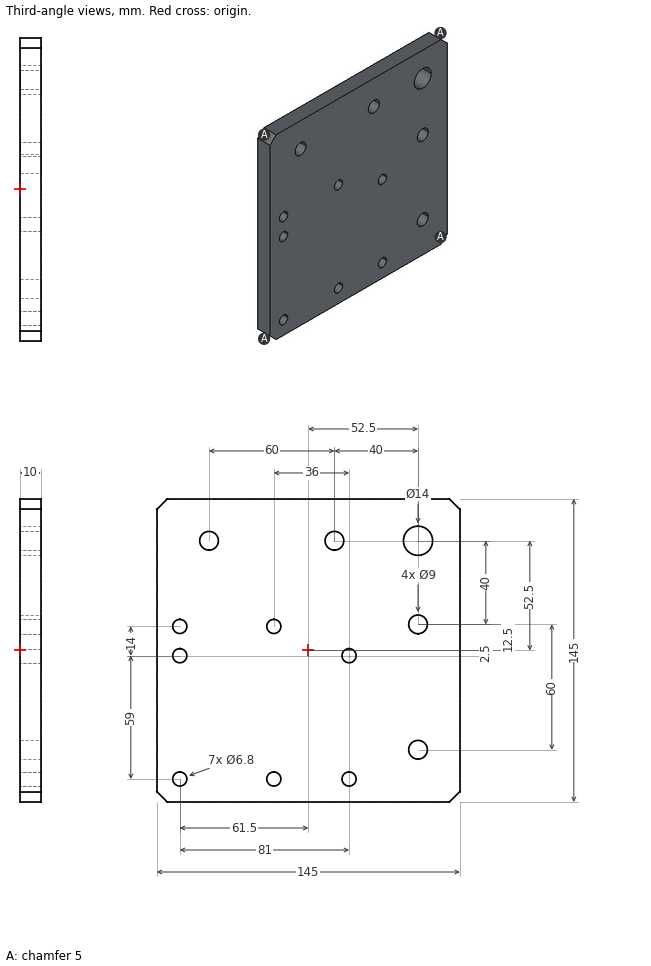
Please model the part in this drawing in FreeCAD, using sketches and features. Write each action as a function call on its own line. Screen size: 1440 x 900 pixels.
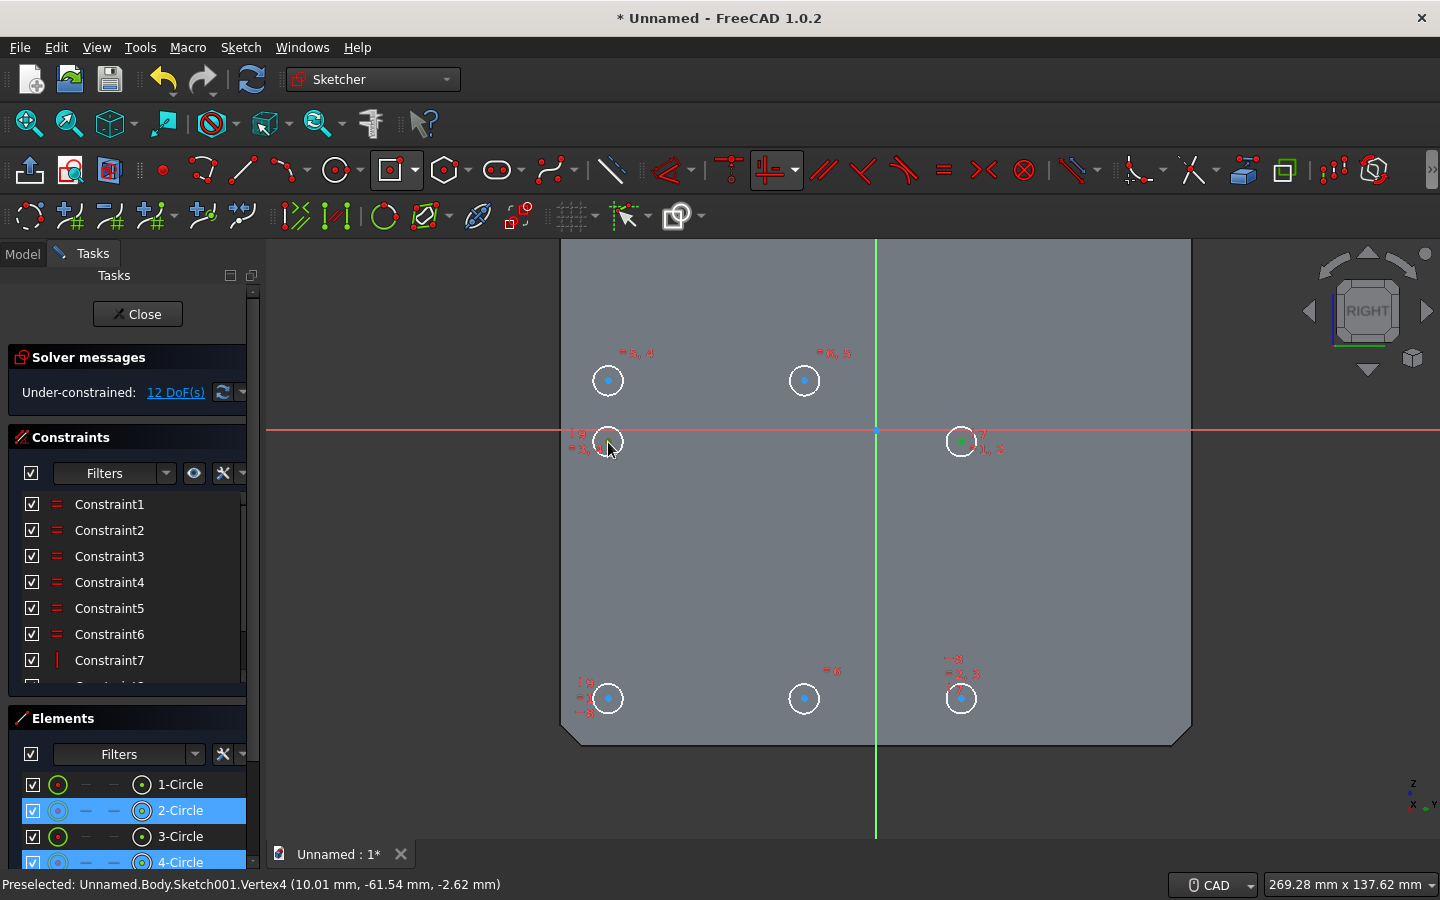
click(798, 170)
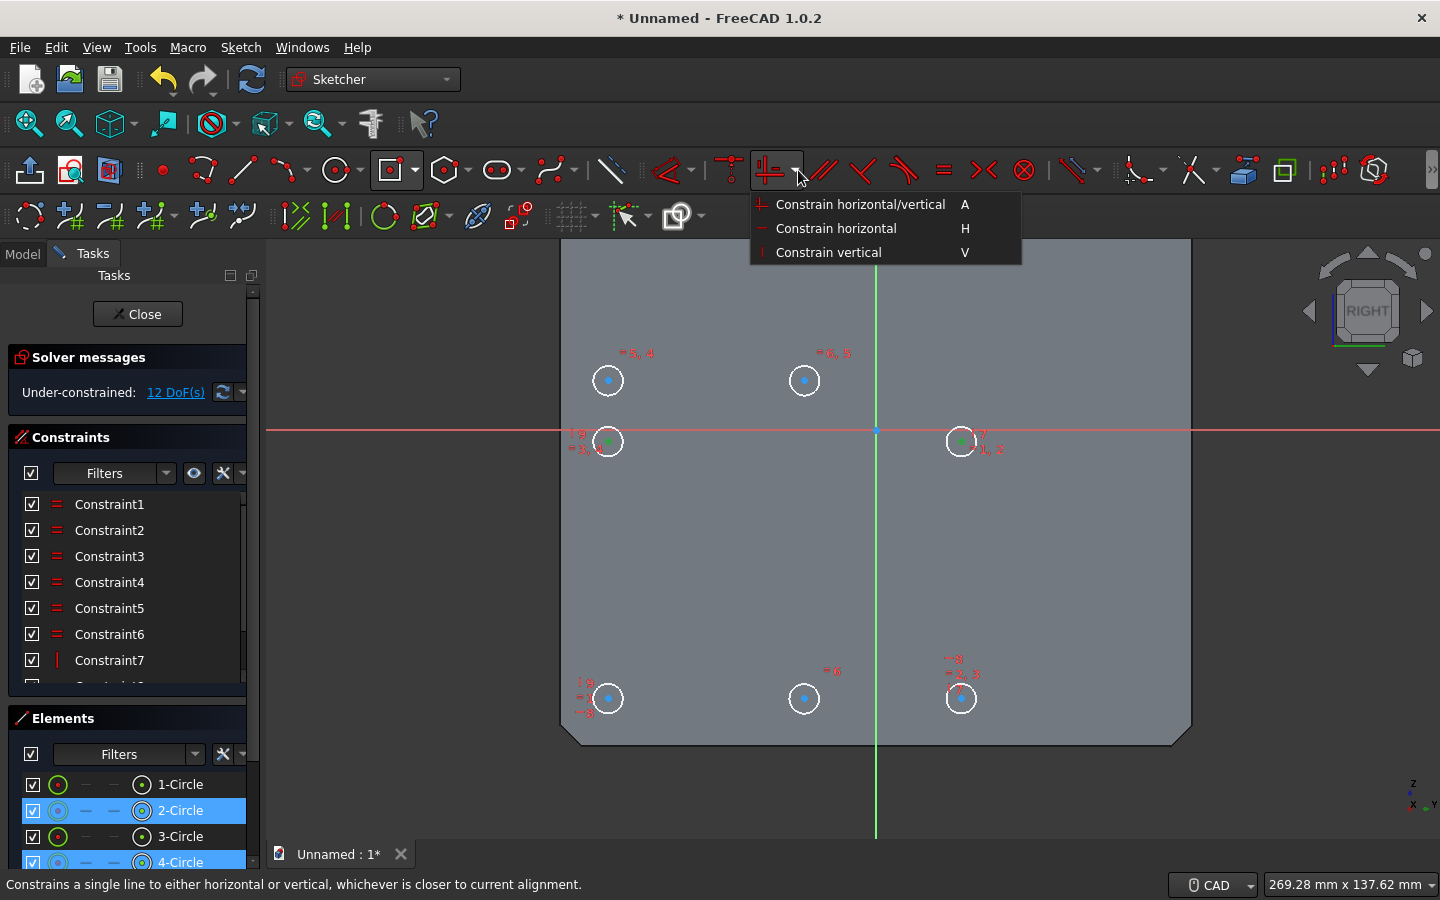
click(886, 228)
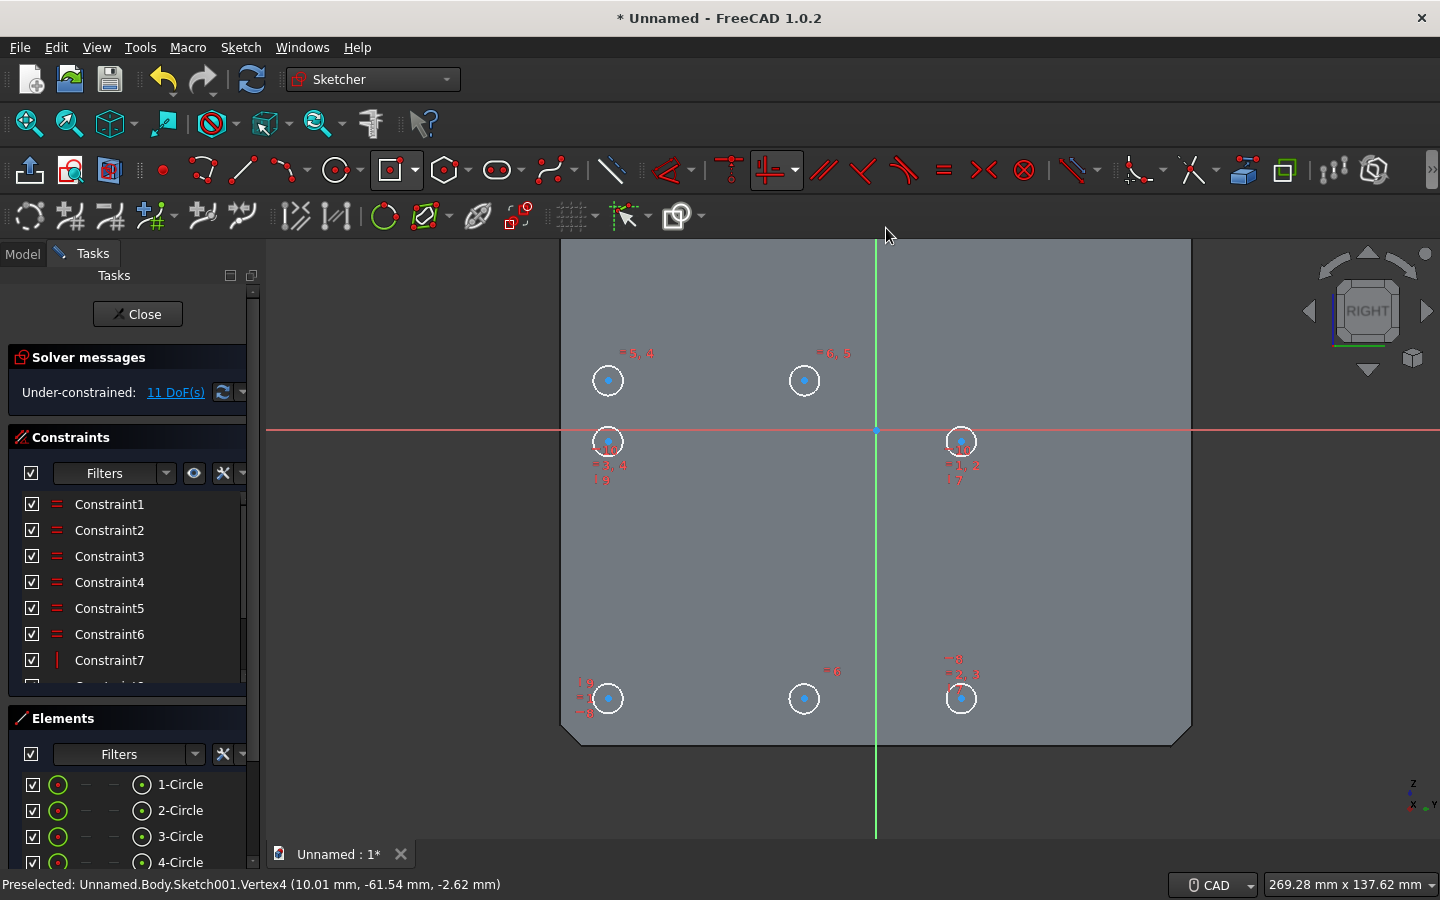
click(608, 442)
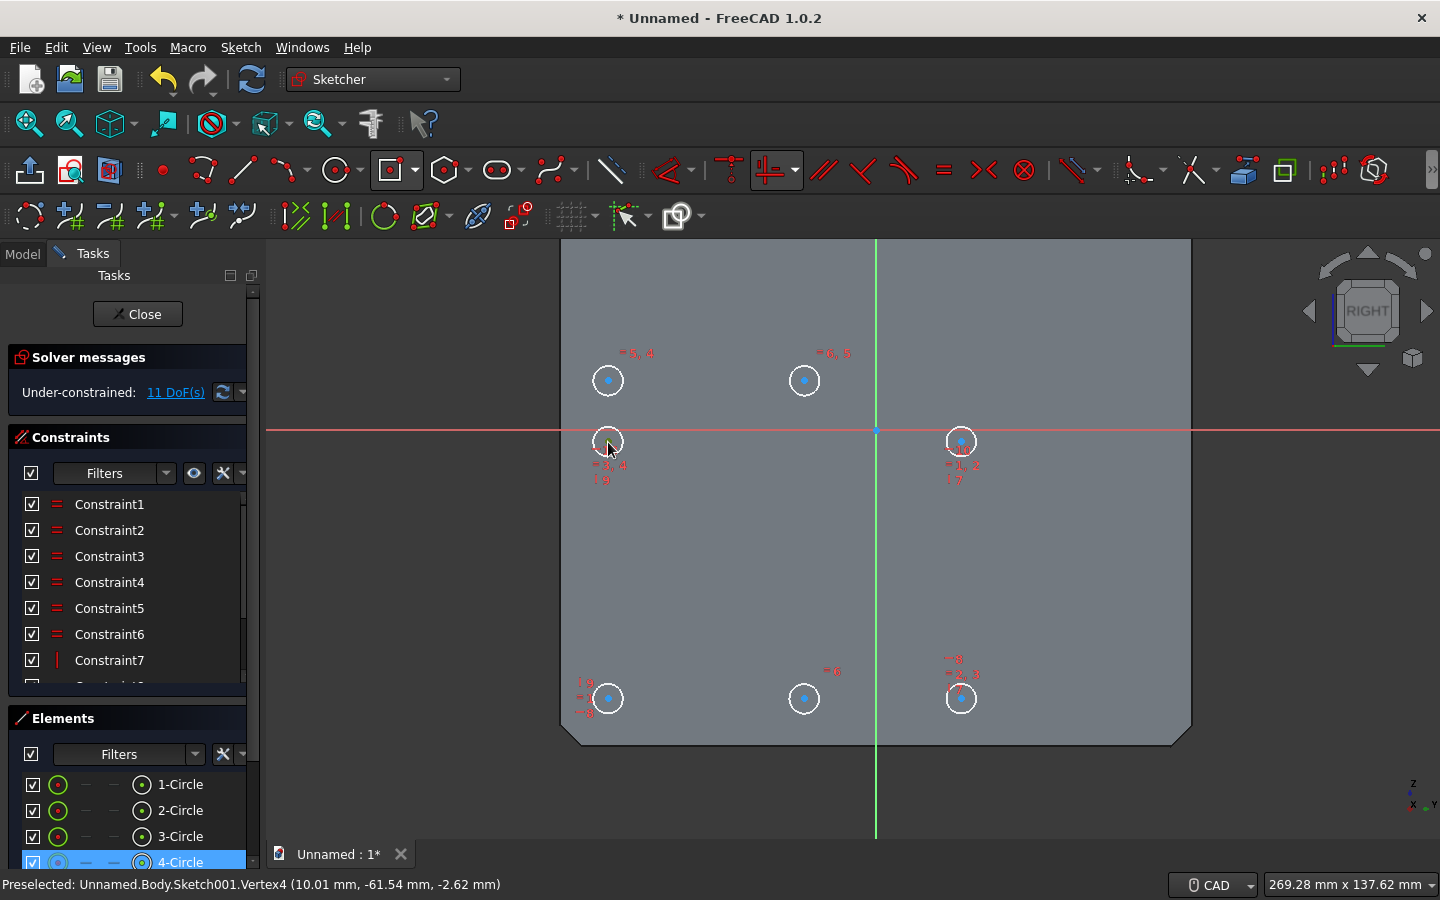
click(608, 381)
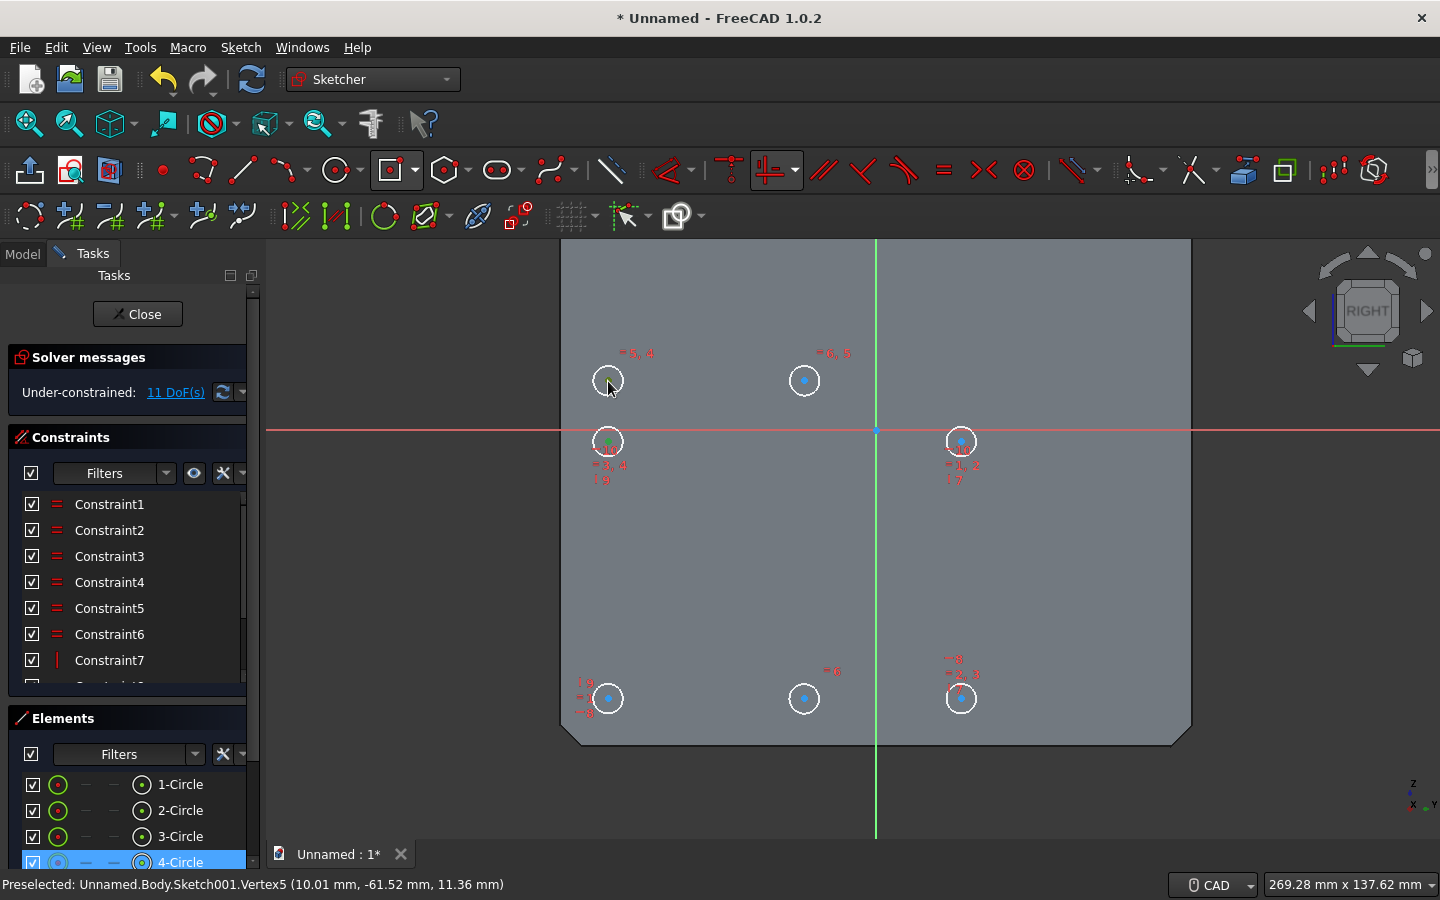
key(v)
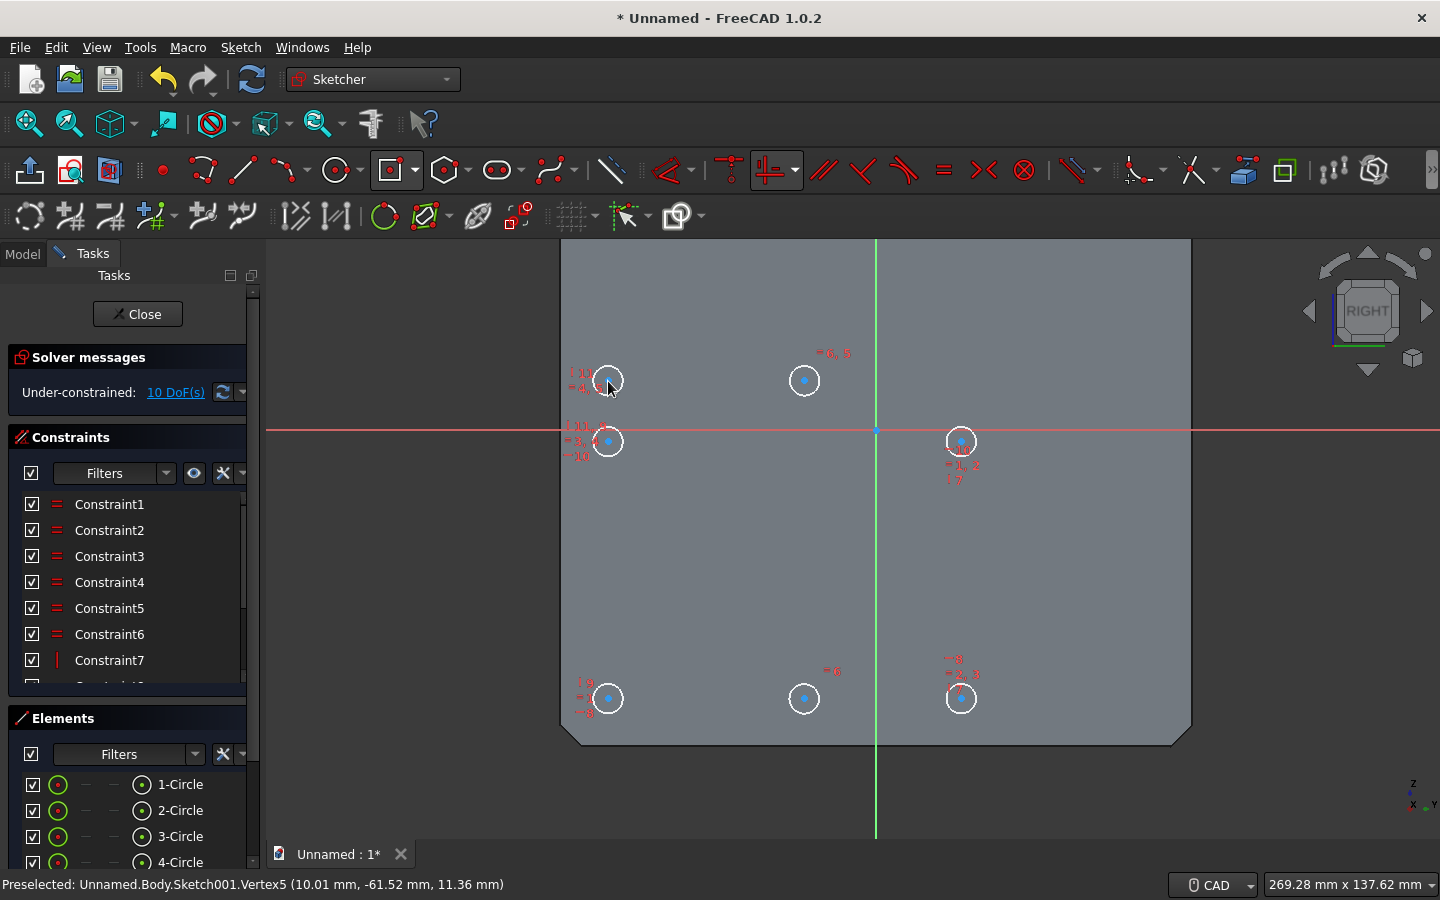
click(608, 381)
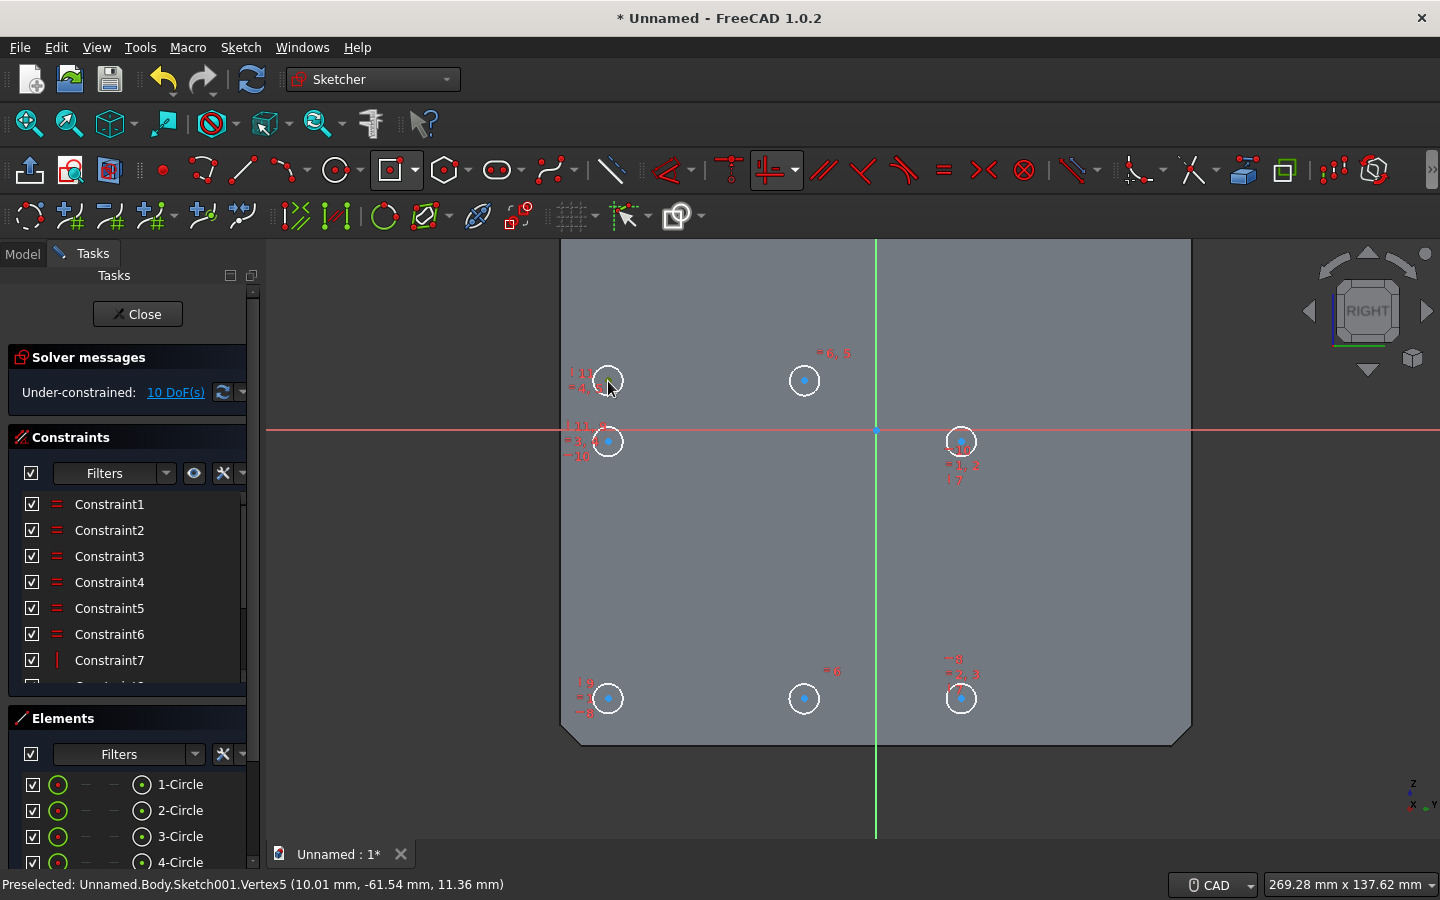
click(805, 381)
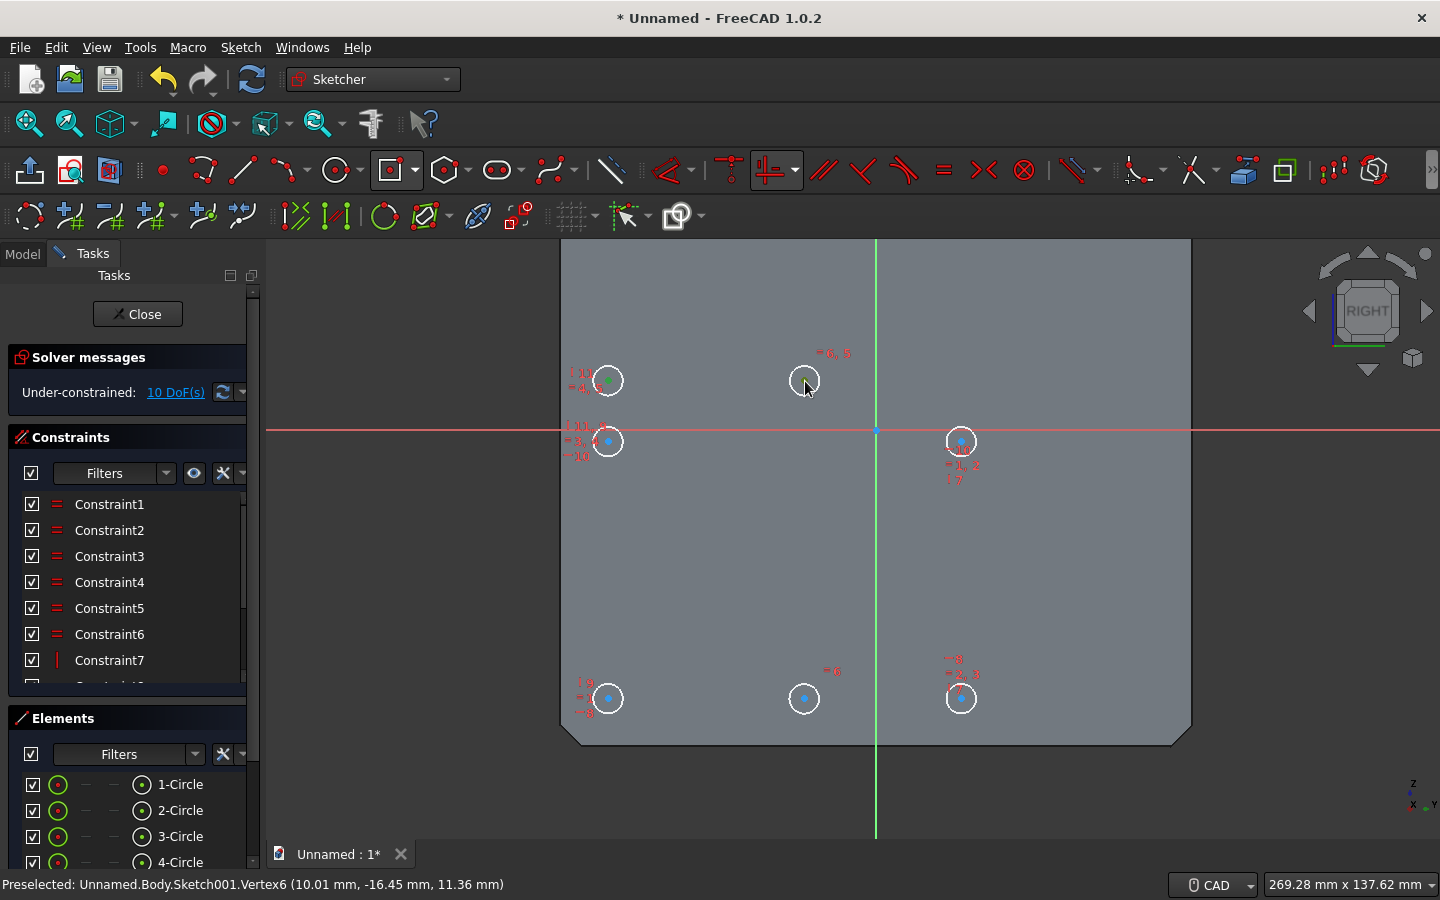
key(h)